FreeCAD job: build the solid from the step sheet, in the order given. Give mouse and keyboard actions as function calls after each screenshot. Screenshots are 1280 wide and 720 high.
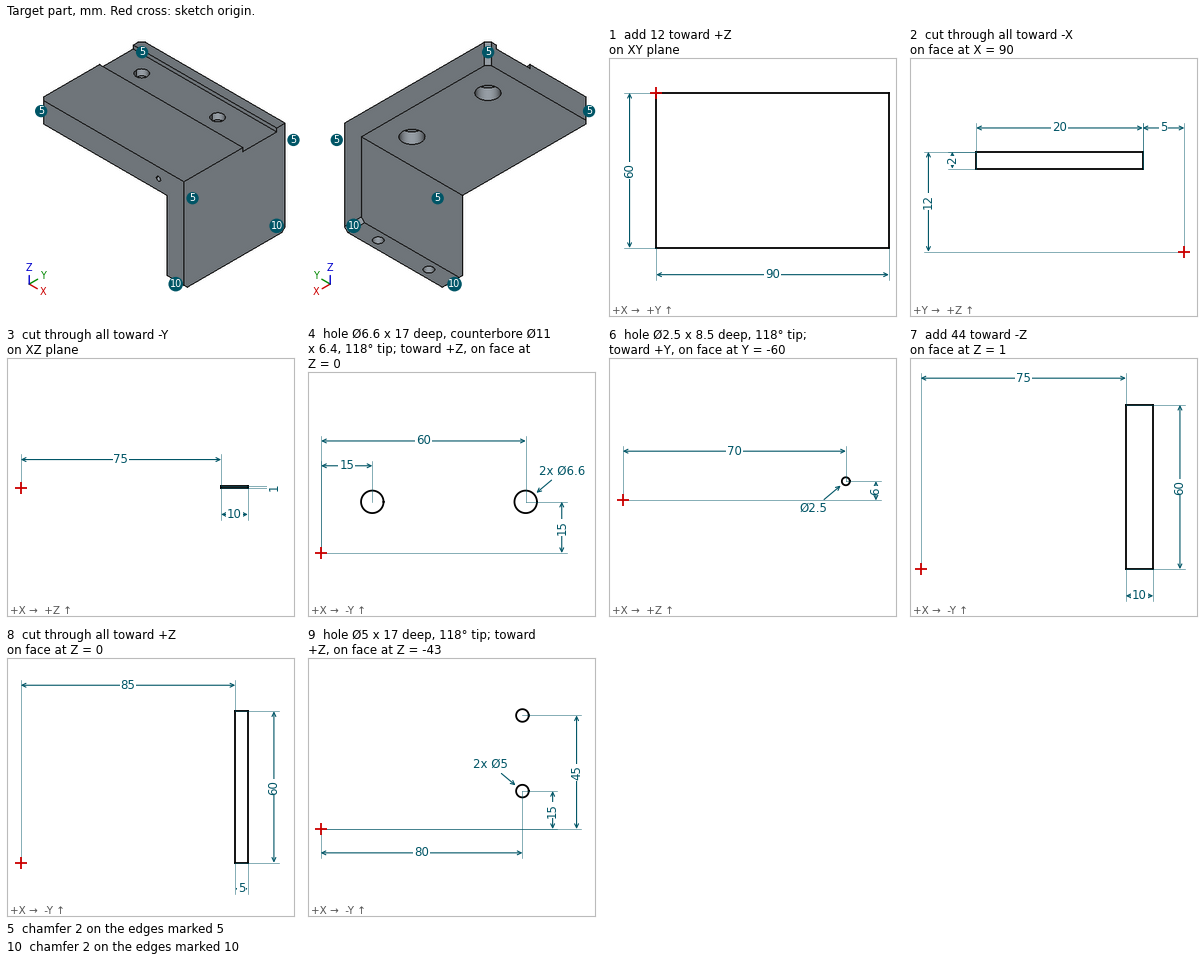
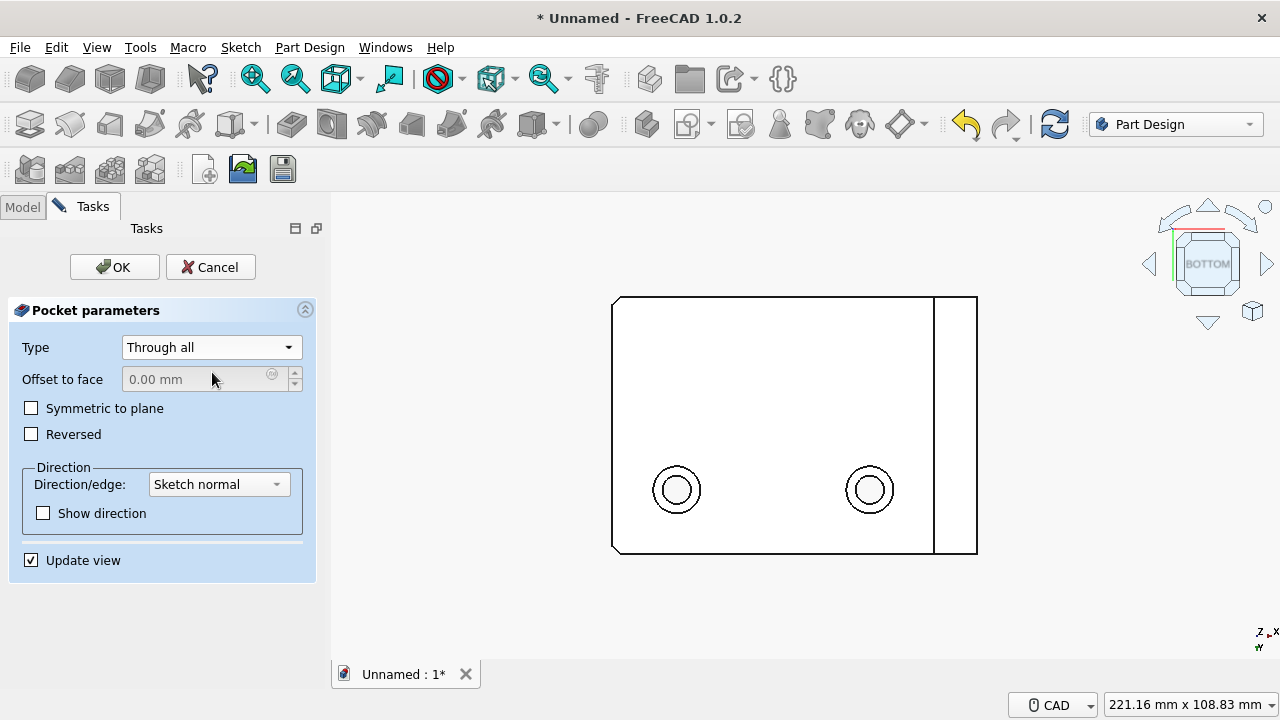
click(115, 267)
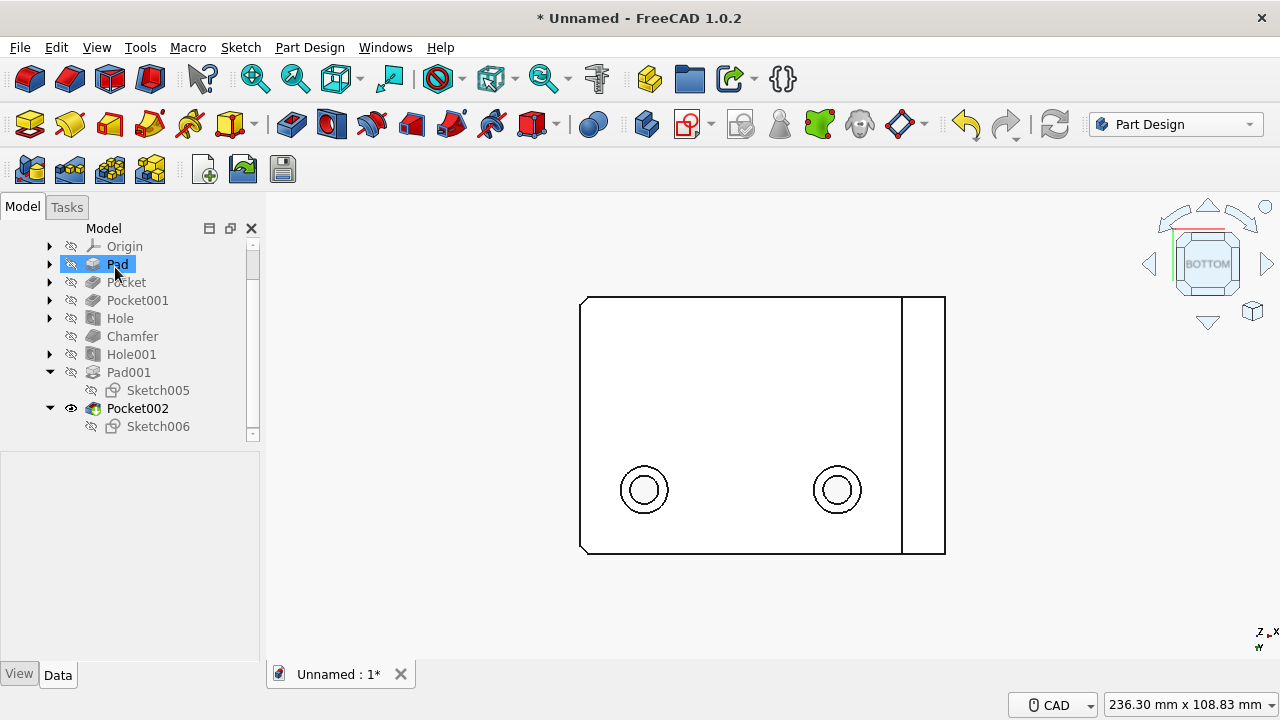
click(923, 498)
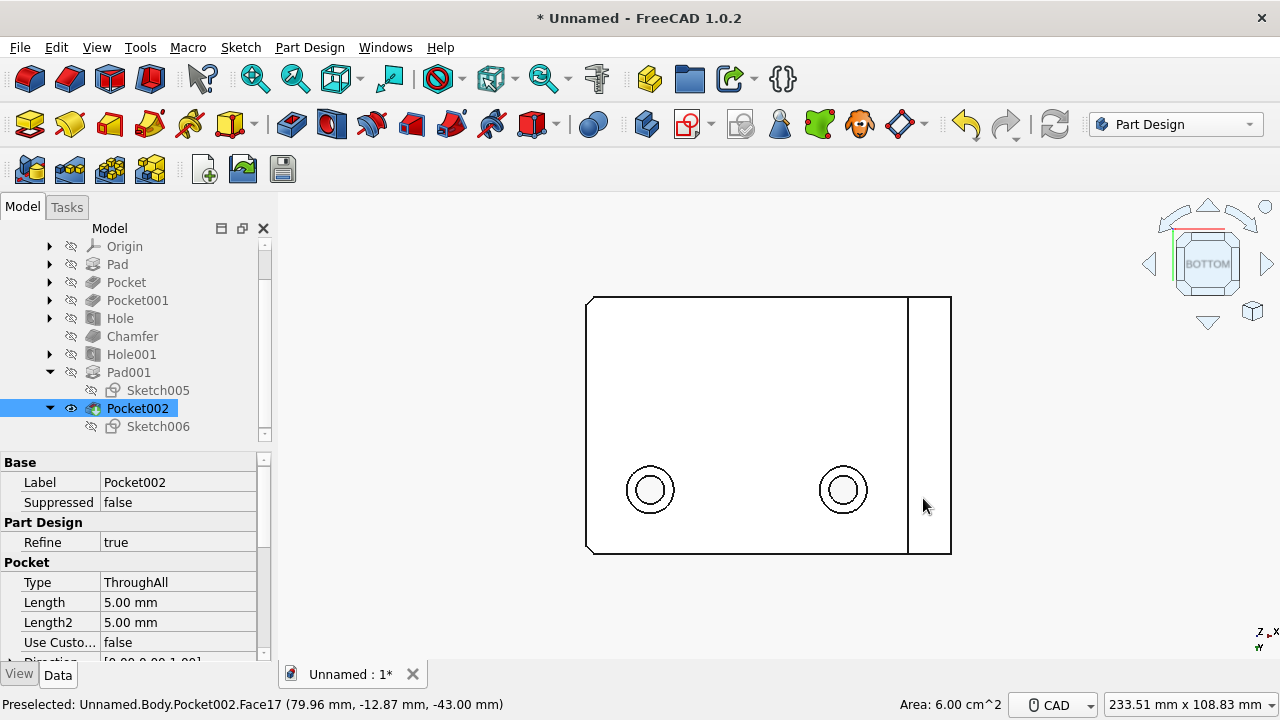
click(688, 124)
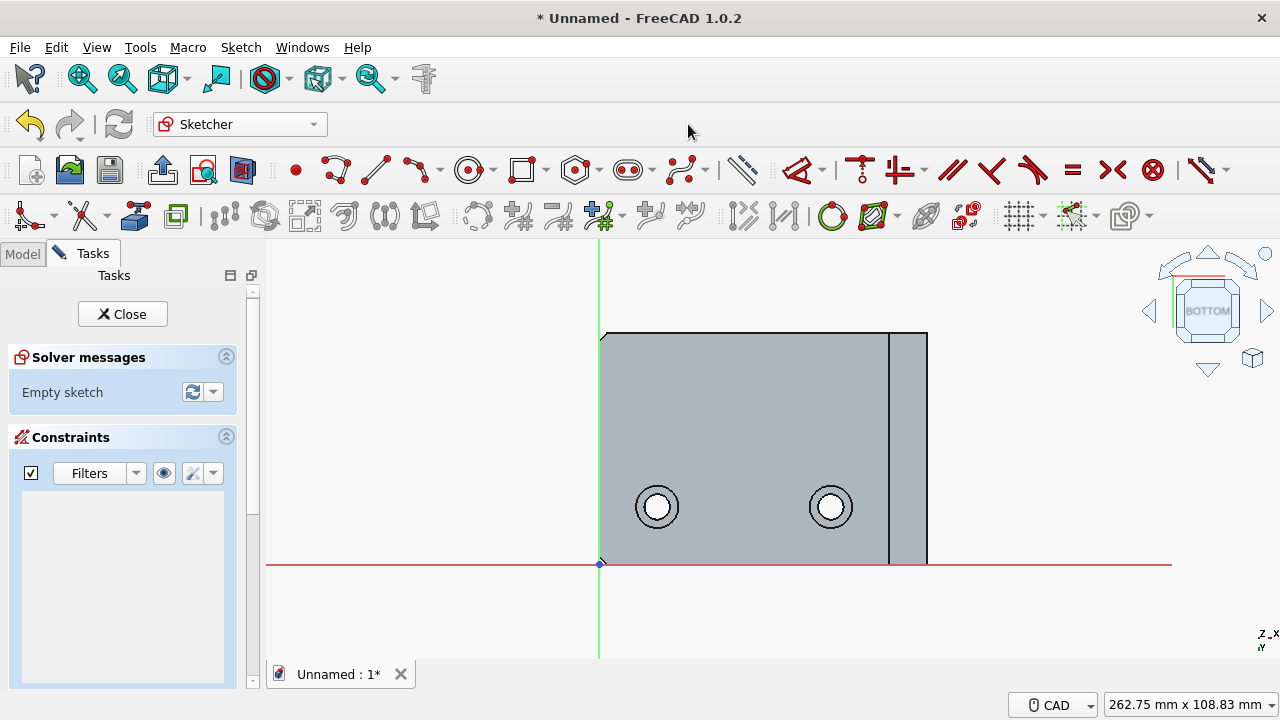
scroll(868, 522, up, 2)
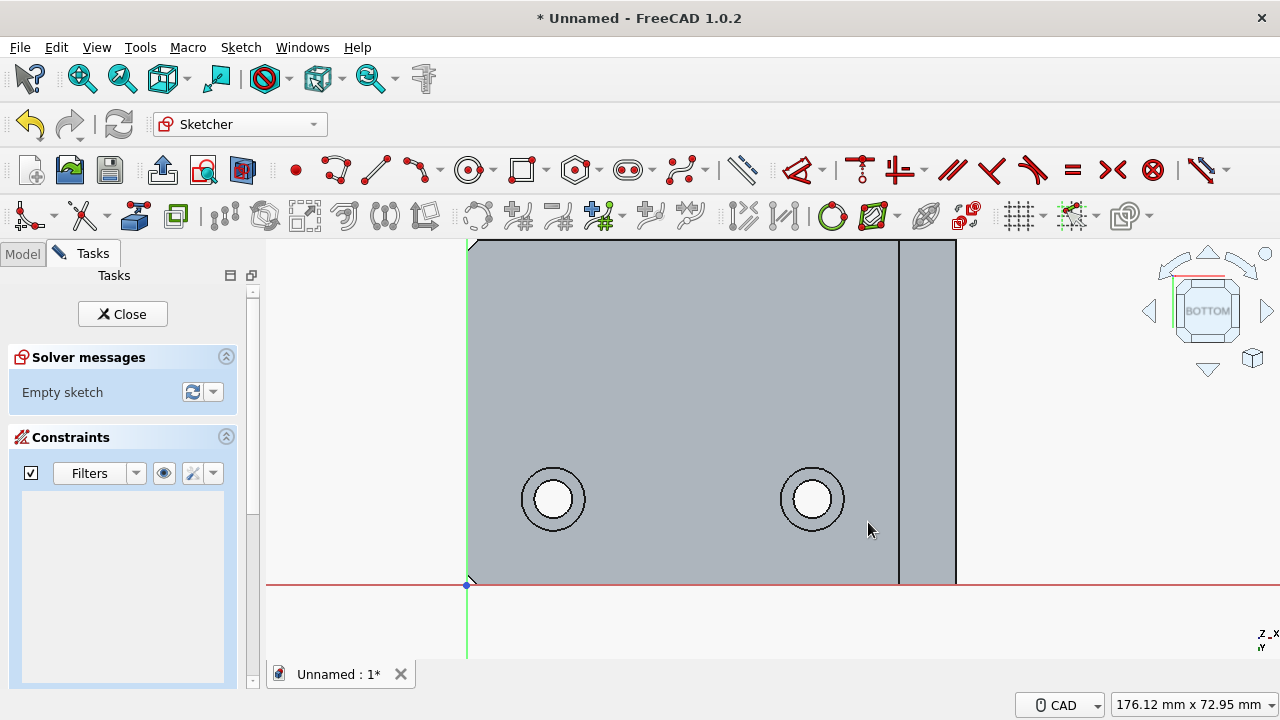
click(470, 170)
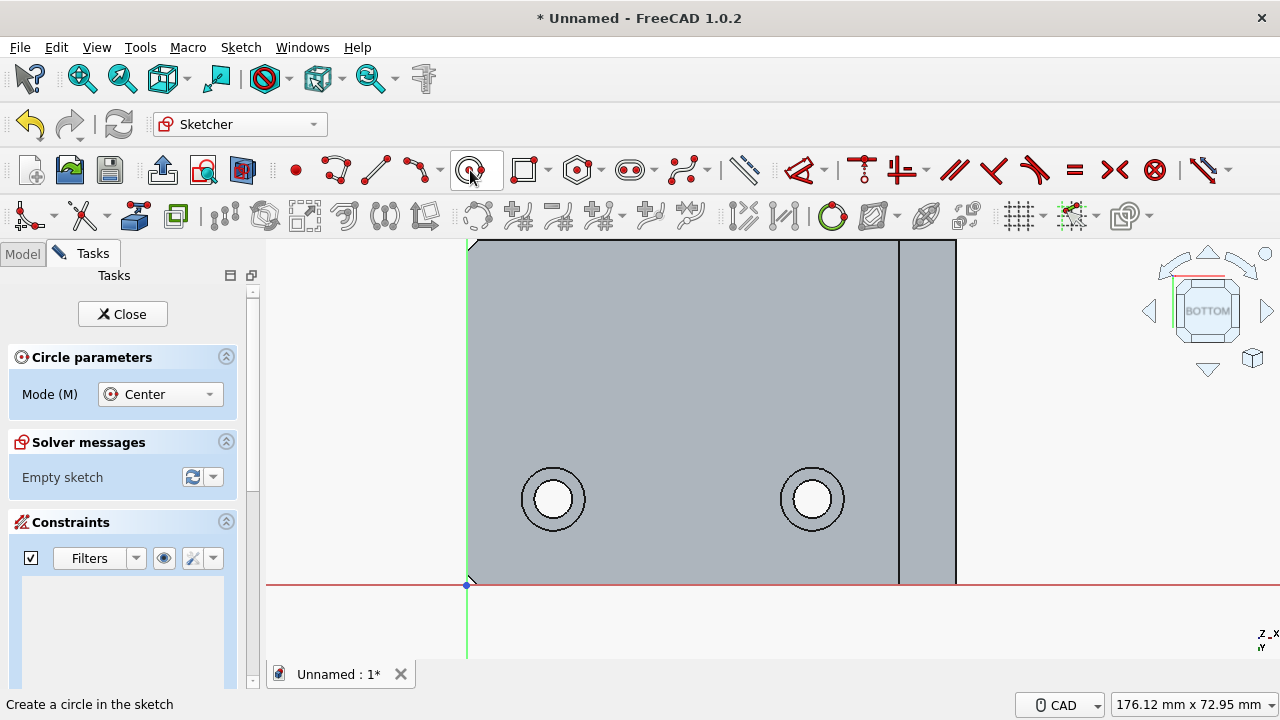
scroll(927, 499, up, 3)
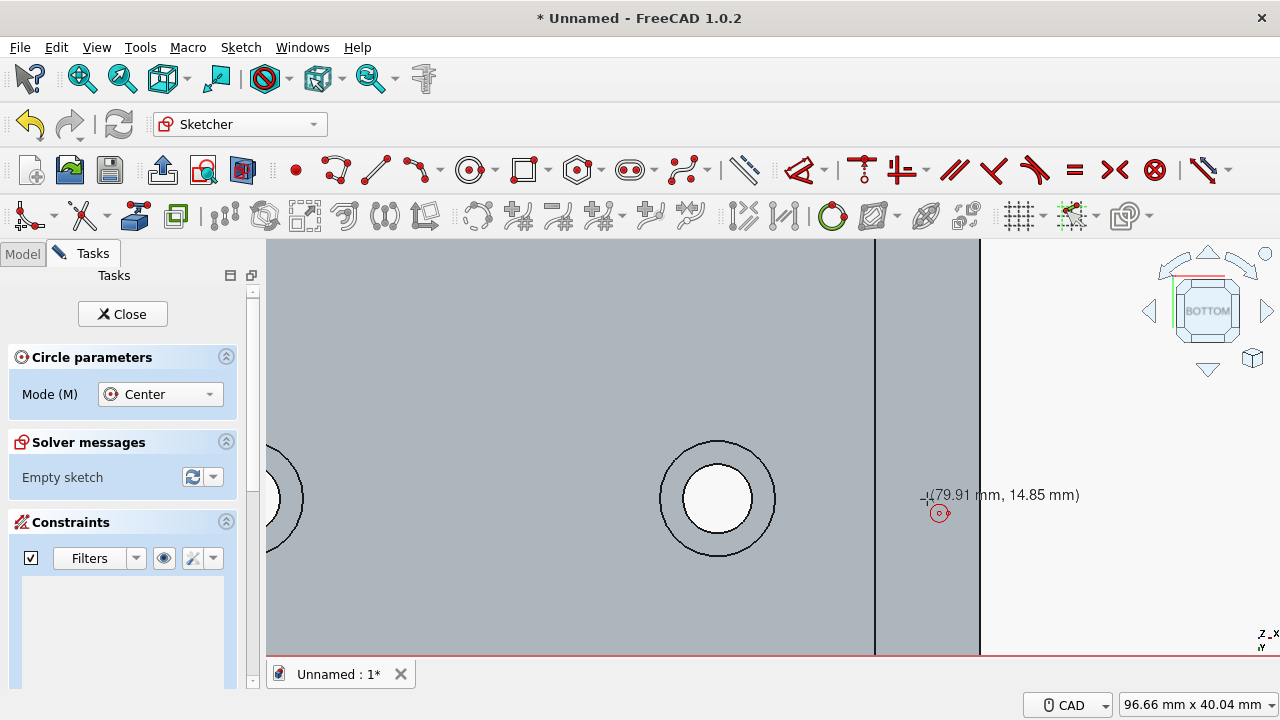
click(927, 499)
click(946, 480)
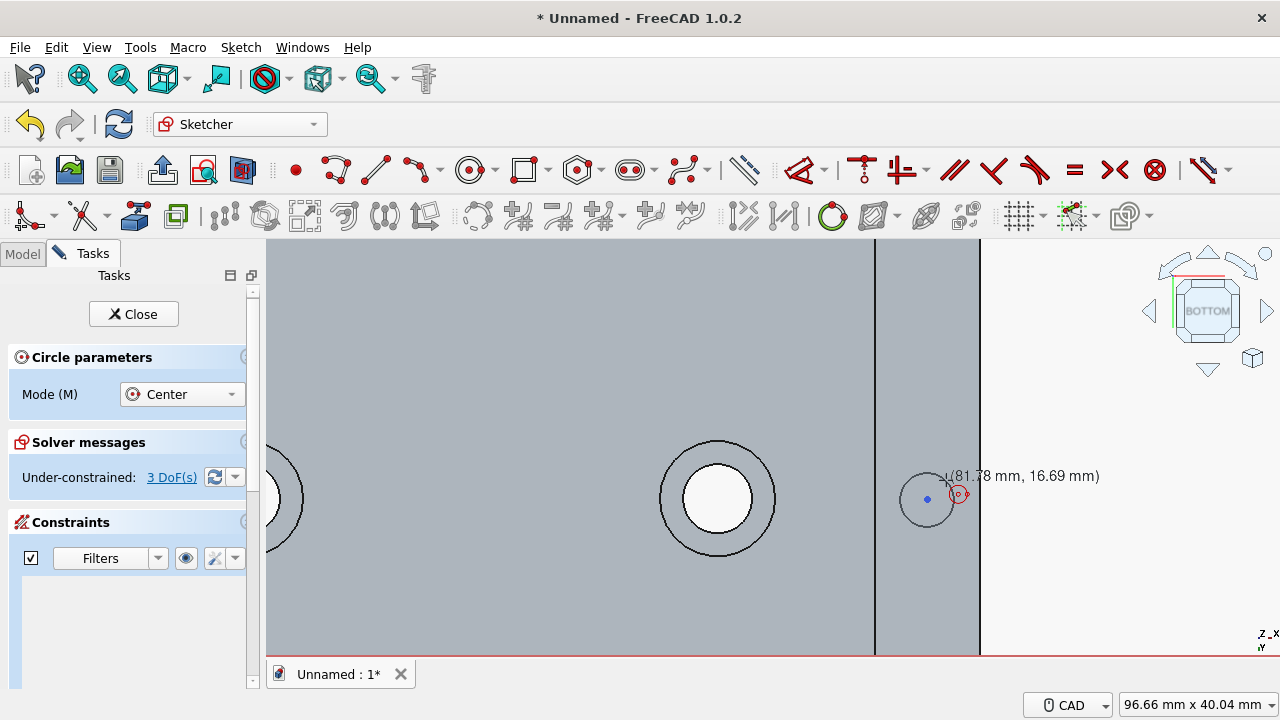
scroll(928, 500, down, 3)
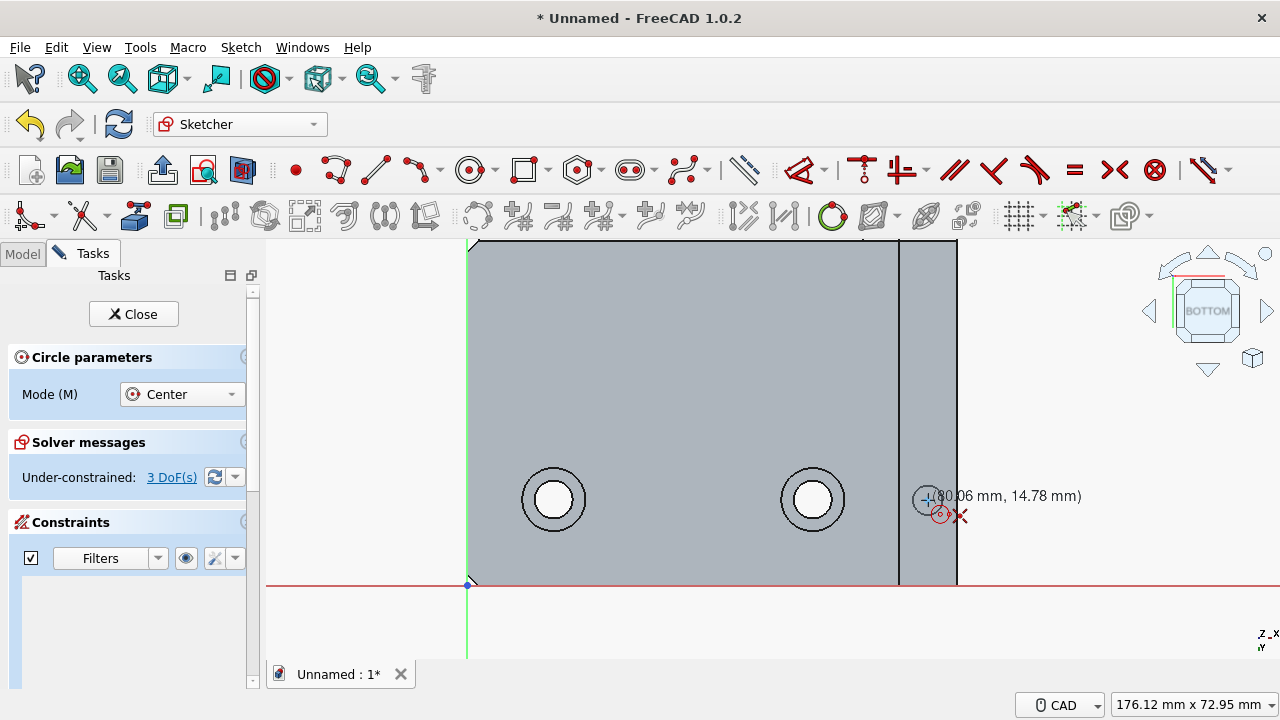
scroll(928, 327, up, 3)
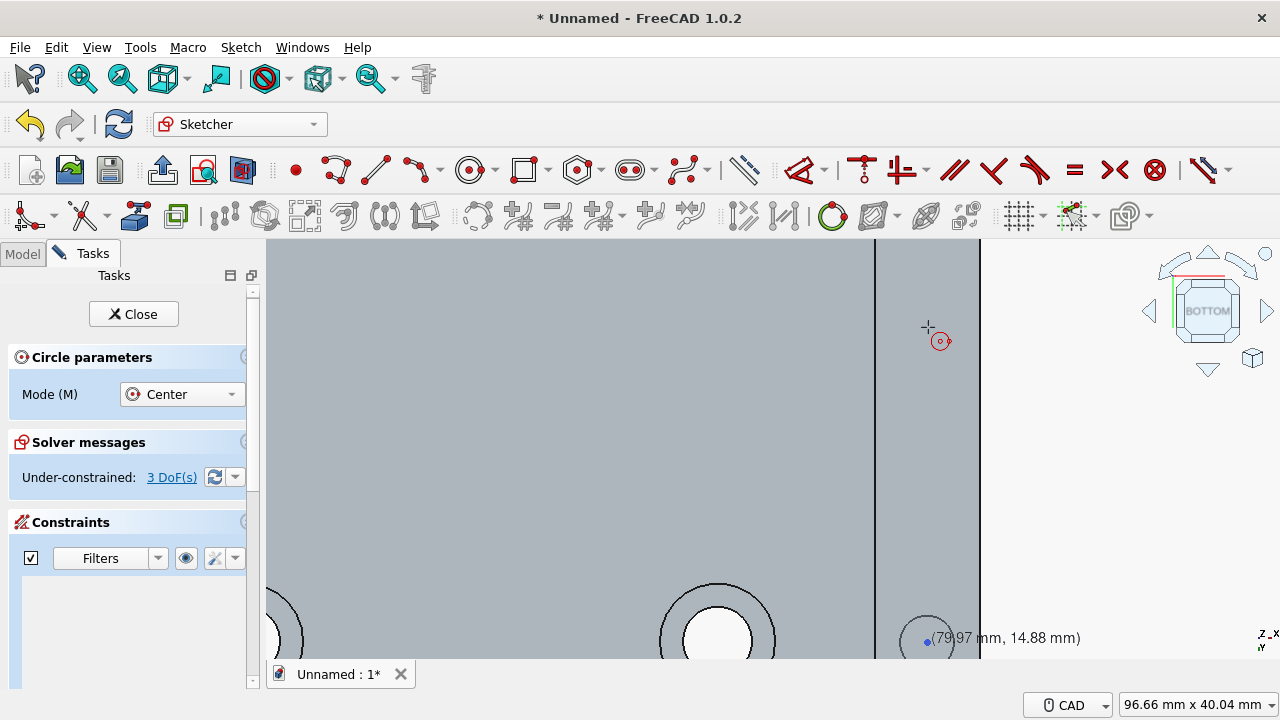
click(927, 327)
click(946, 308)
key(Escape)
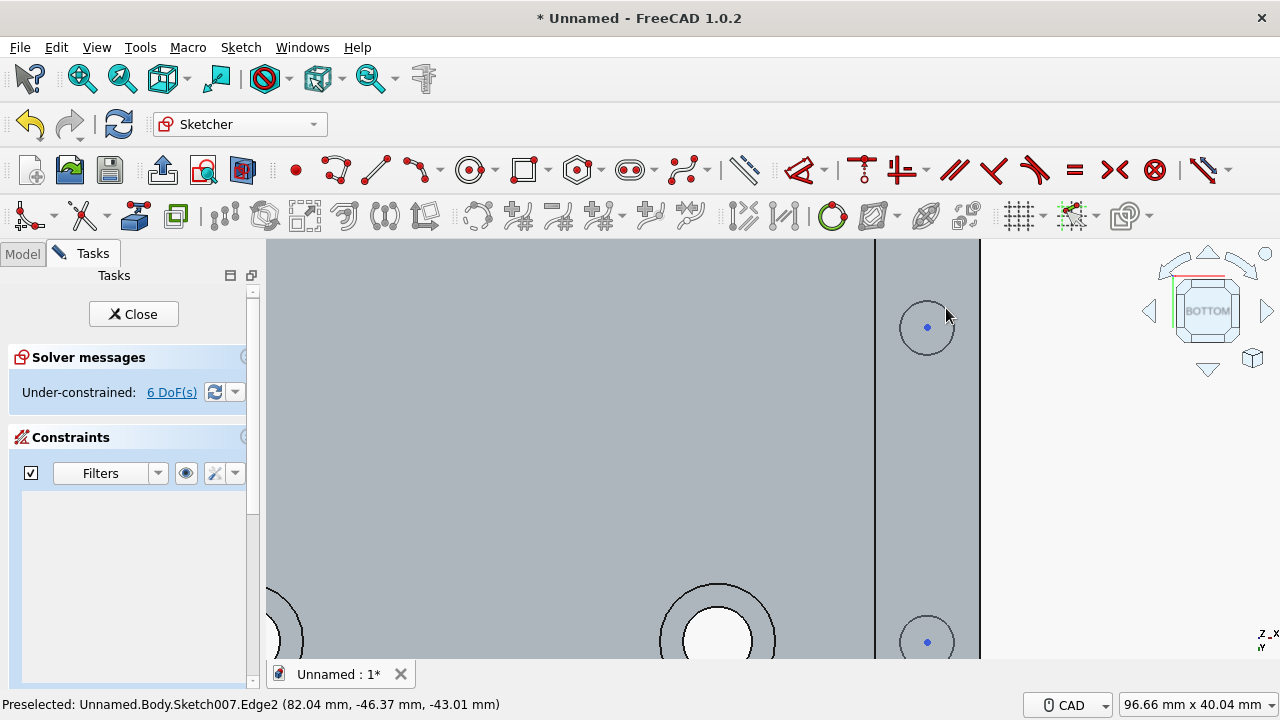
click(946, 624)